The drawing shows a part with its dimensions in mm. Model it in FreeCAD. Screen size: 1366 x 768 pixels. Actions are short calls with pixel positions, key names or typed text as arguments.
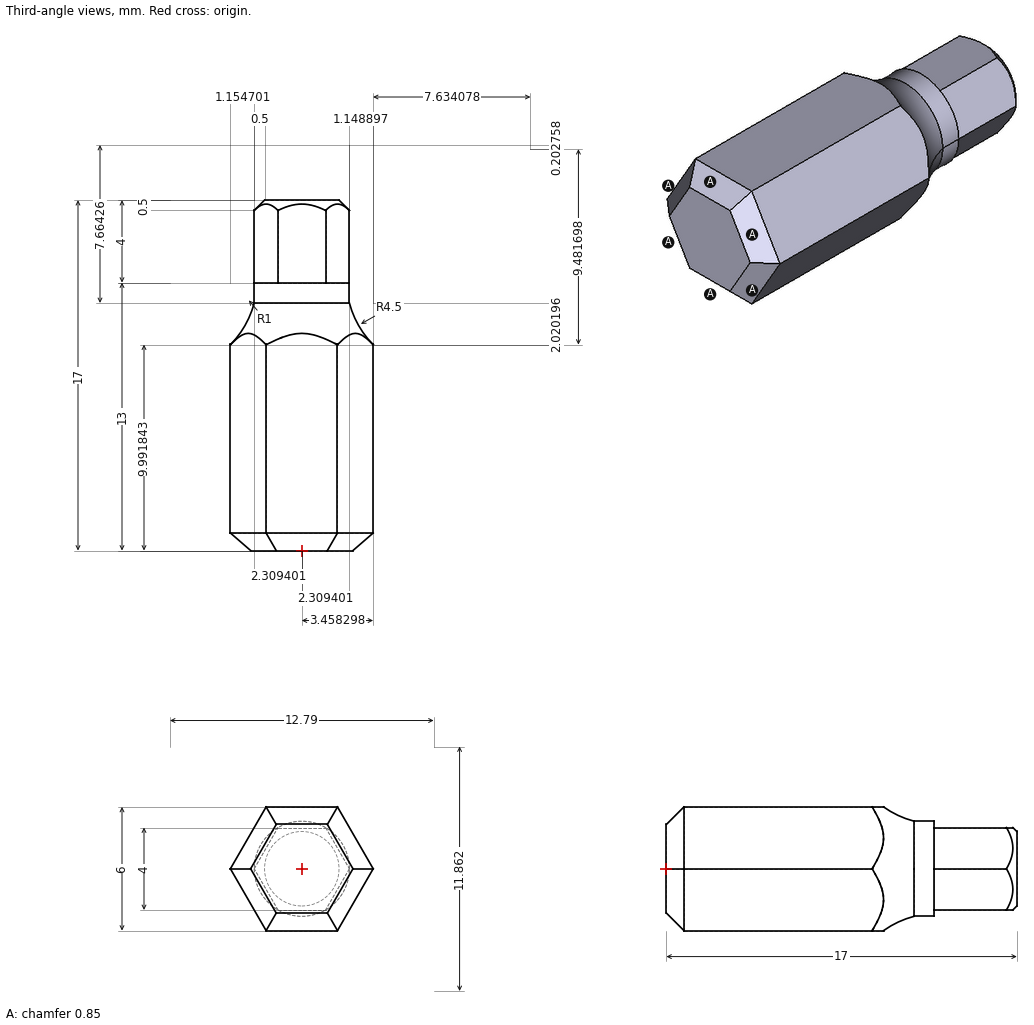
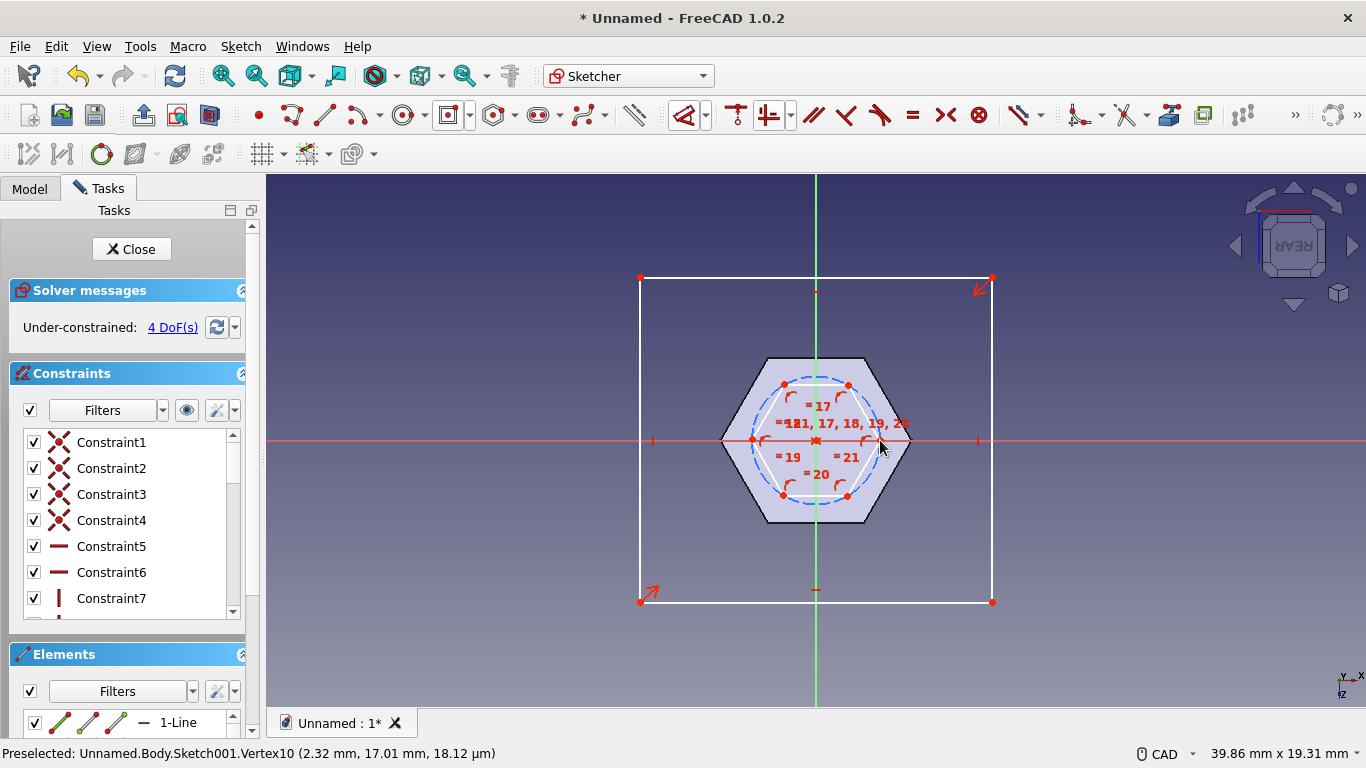
scroll(816, 385, up, 3)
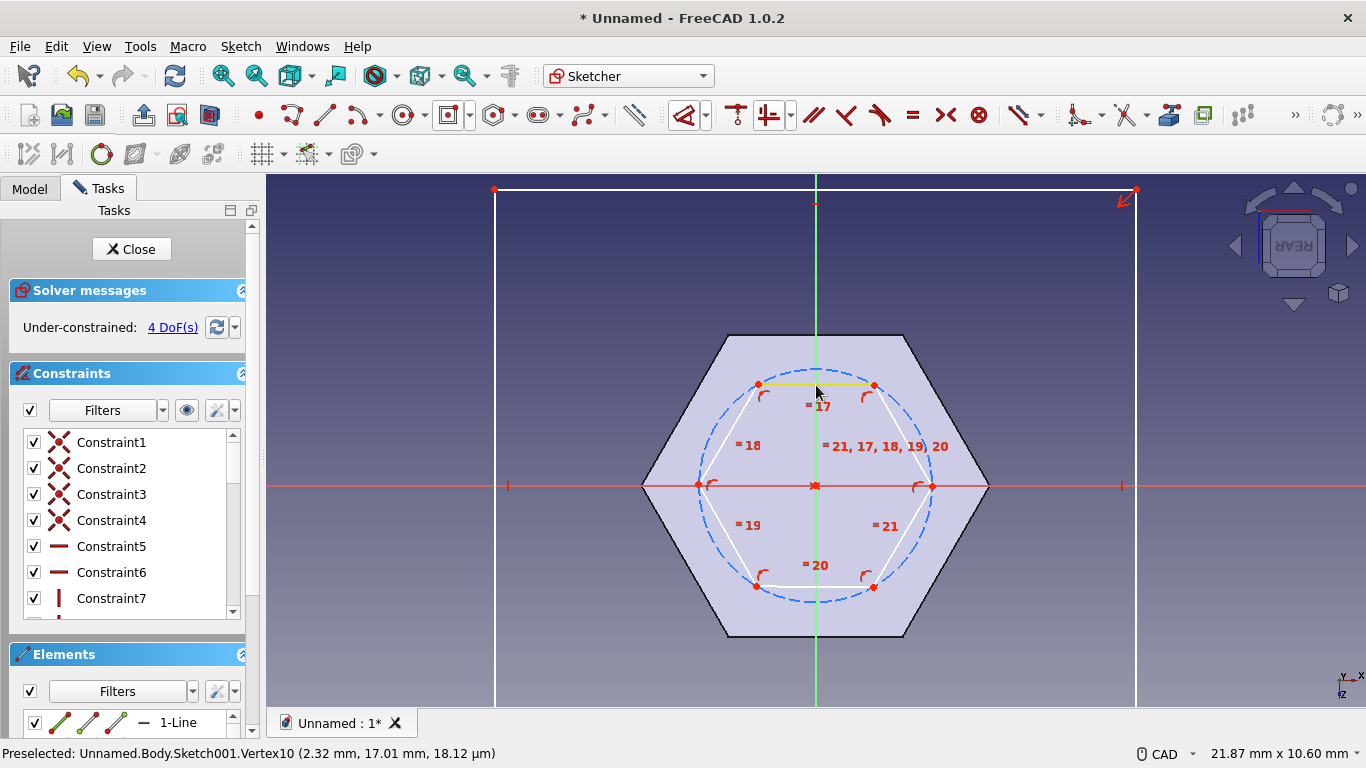
click(816, 385)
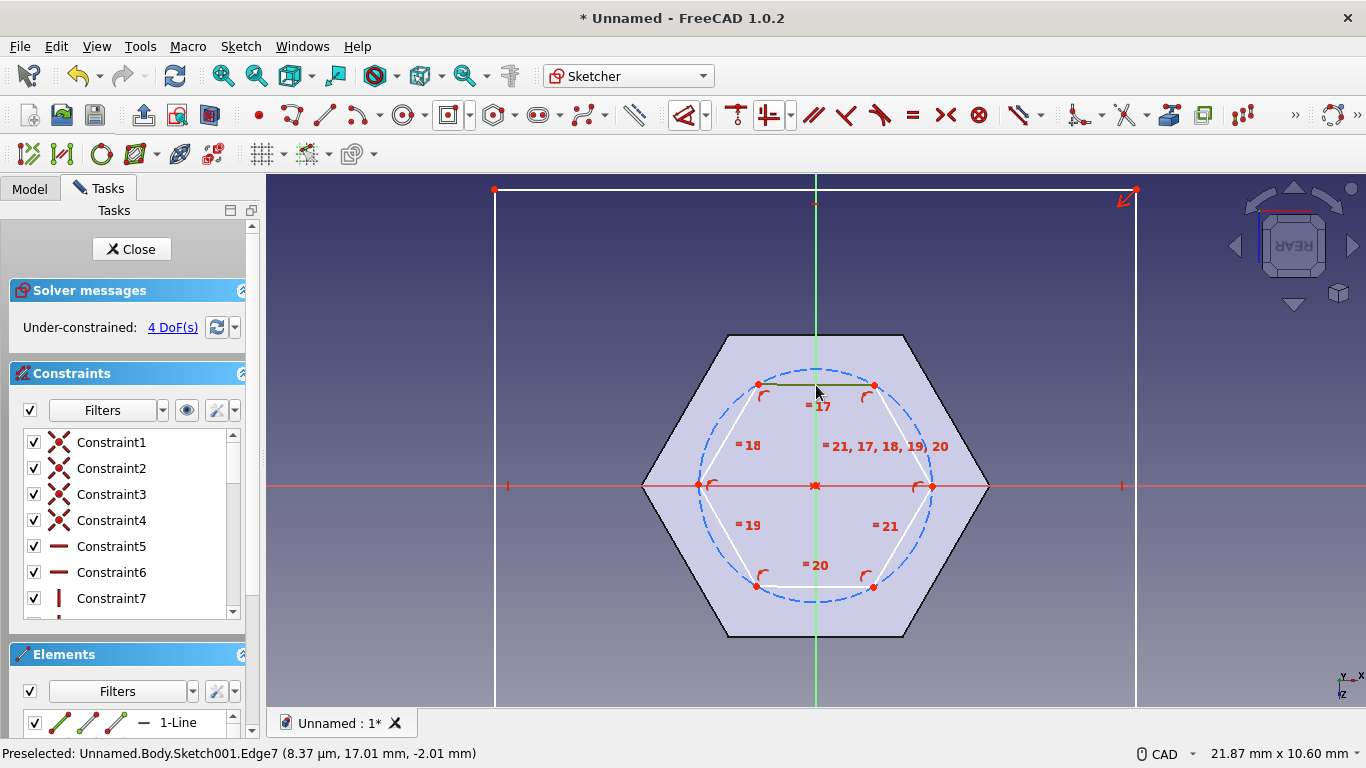
key(h)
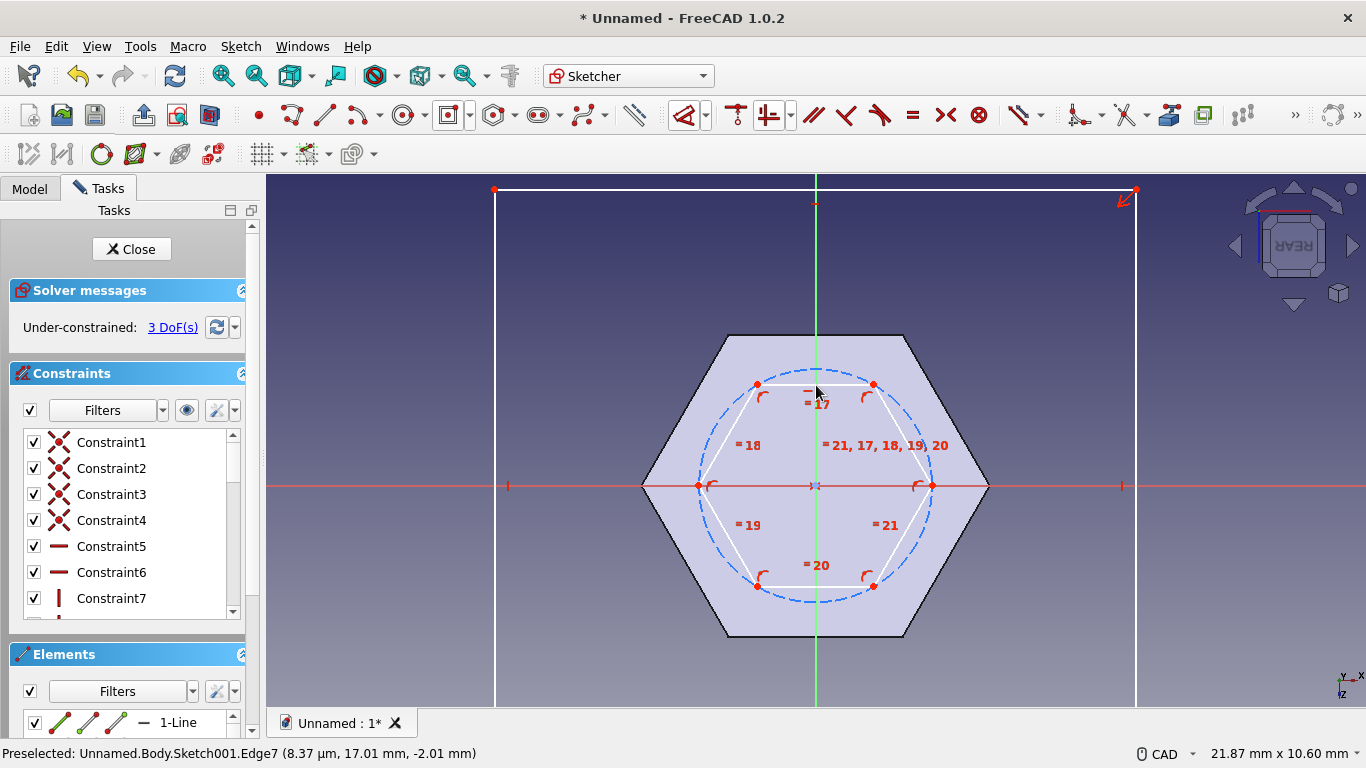
click(757, 587)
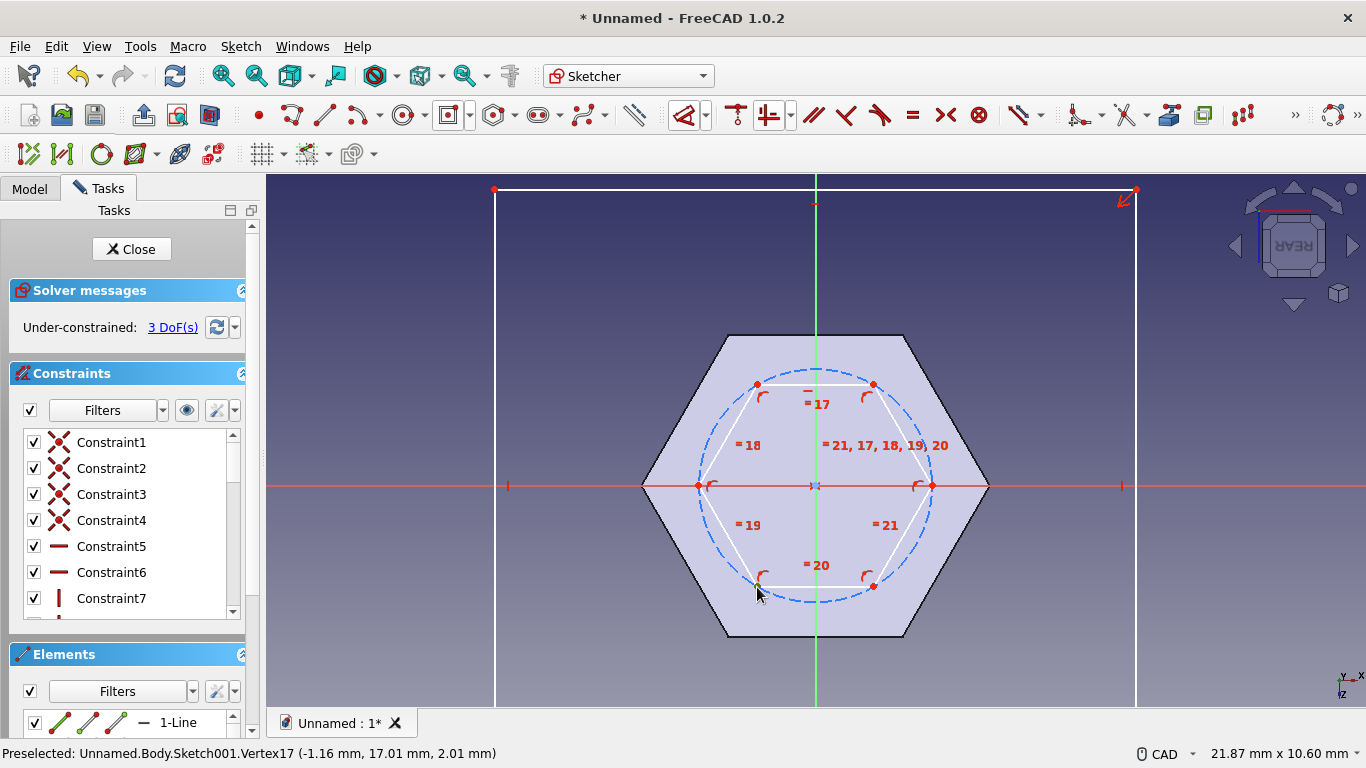
click(874, 385)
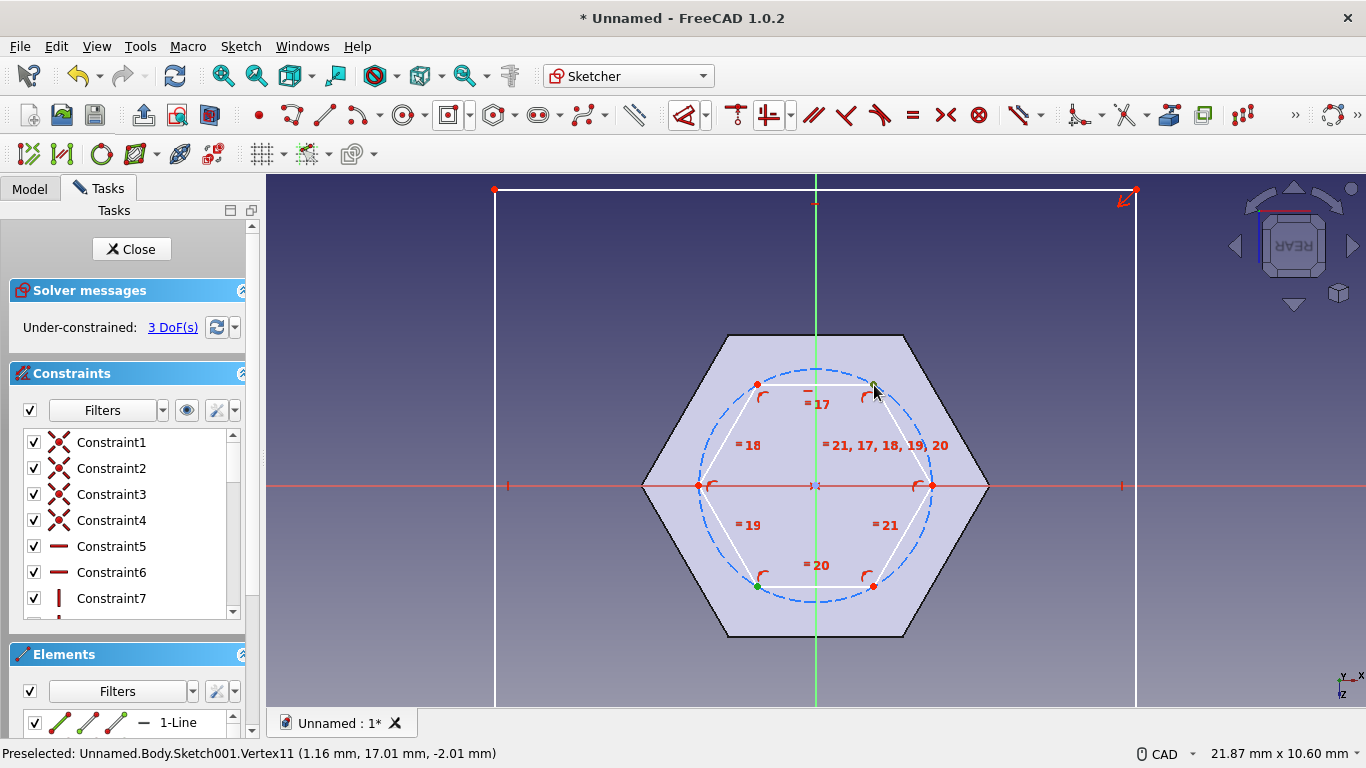
click(706, 116)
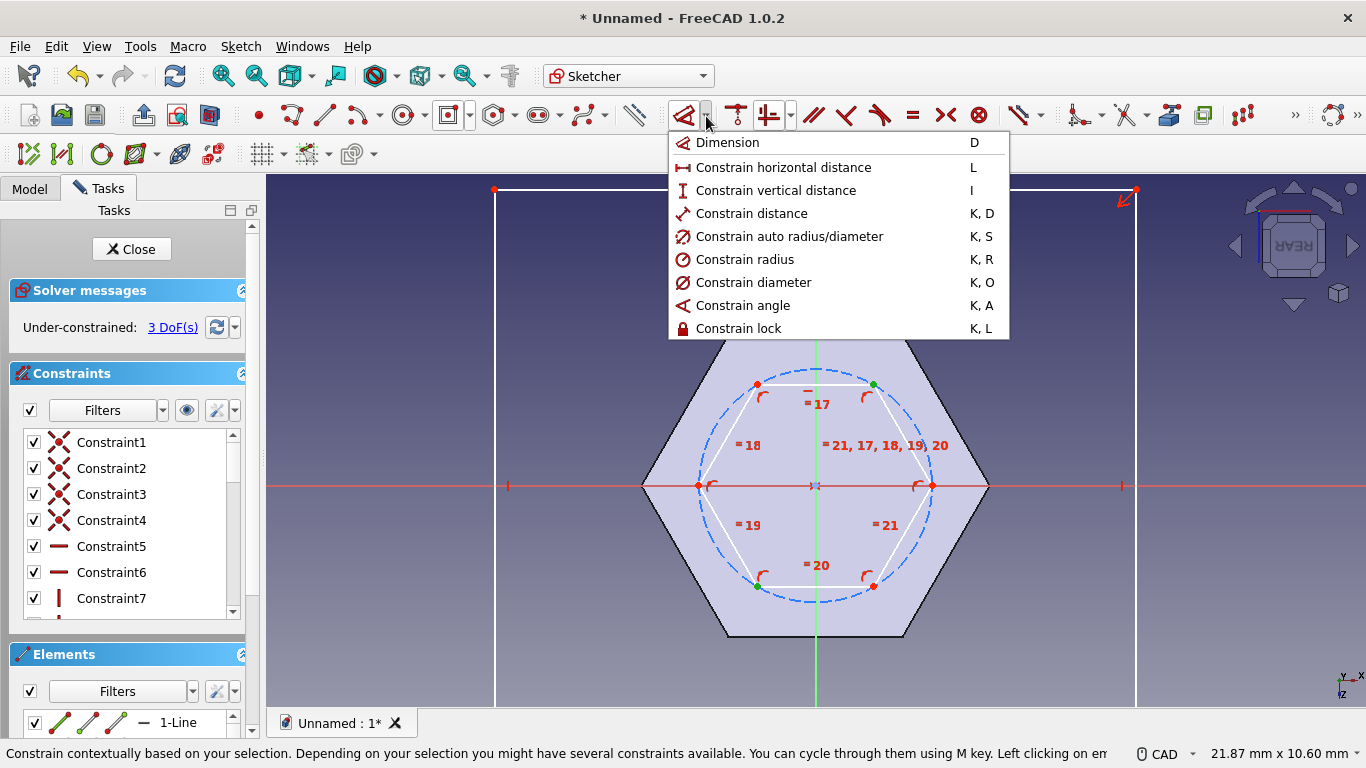
click(839, 190)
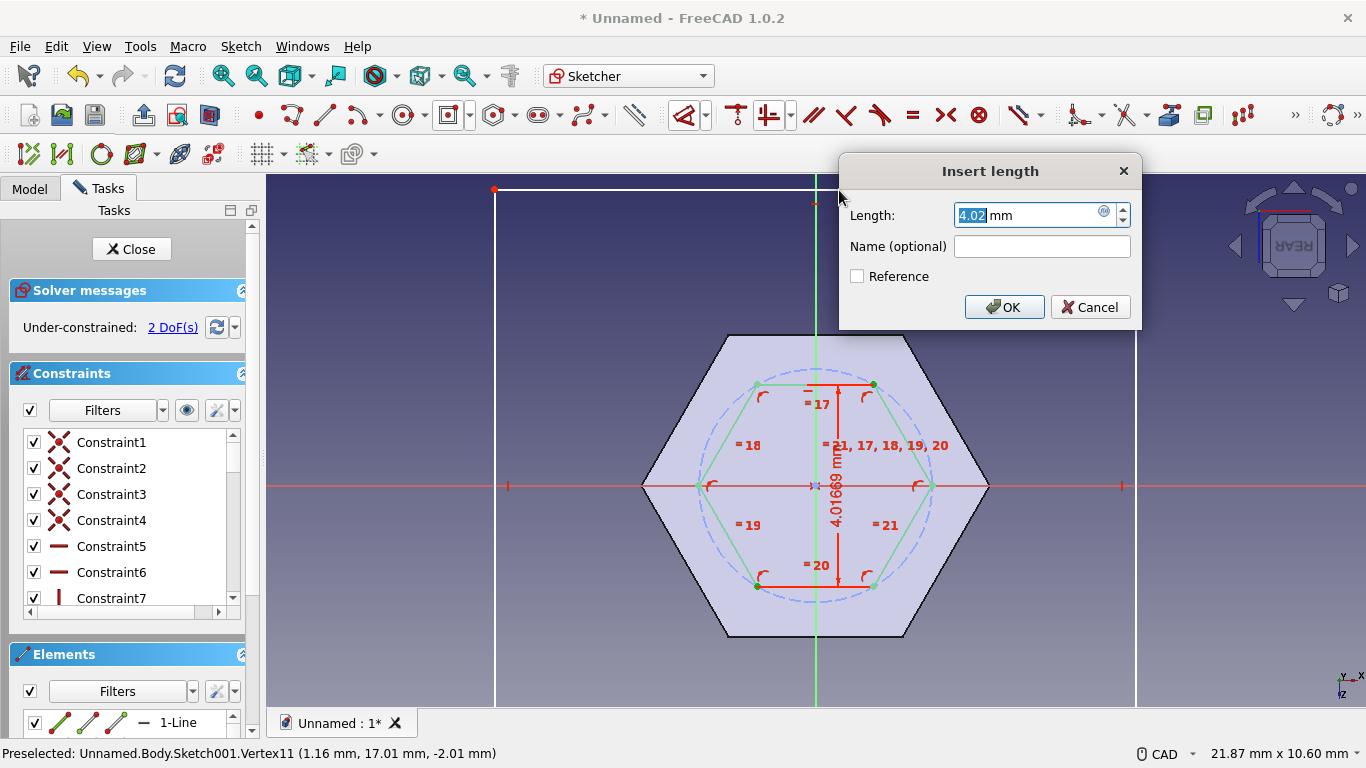
text(4)
key(Return)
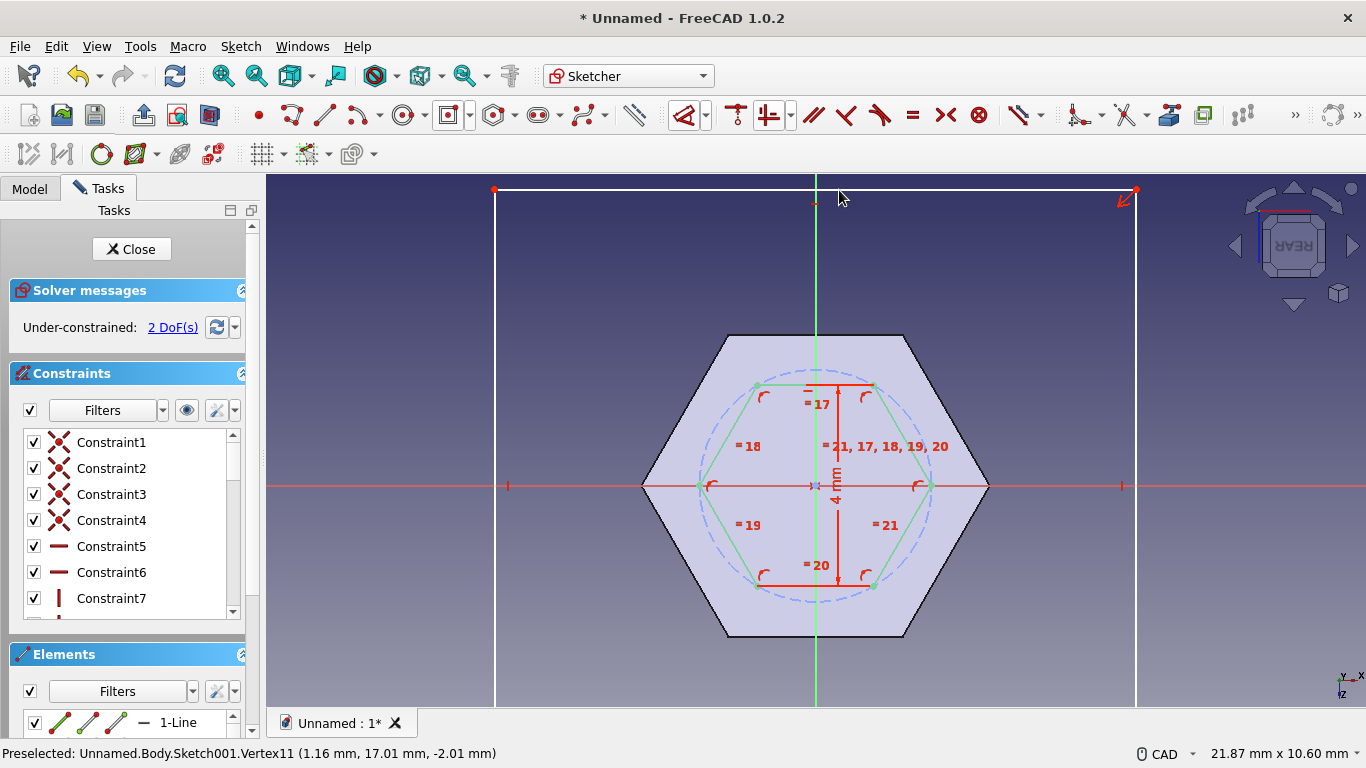
scroll(665, 385, down, 3)